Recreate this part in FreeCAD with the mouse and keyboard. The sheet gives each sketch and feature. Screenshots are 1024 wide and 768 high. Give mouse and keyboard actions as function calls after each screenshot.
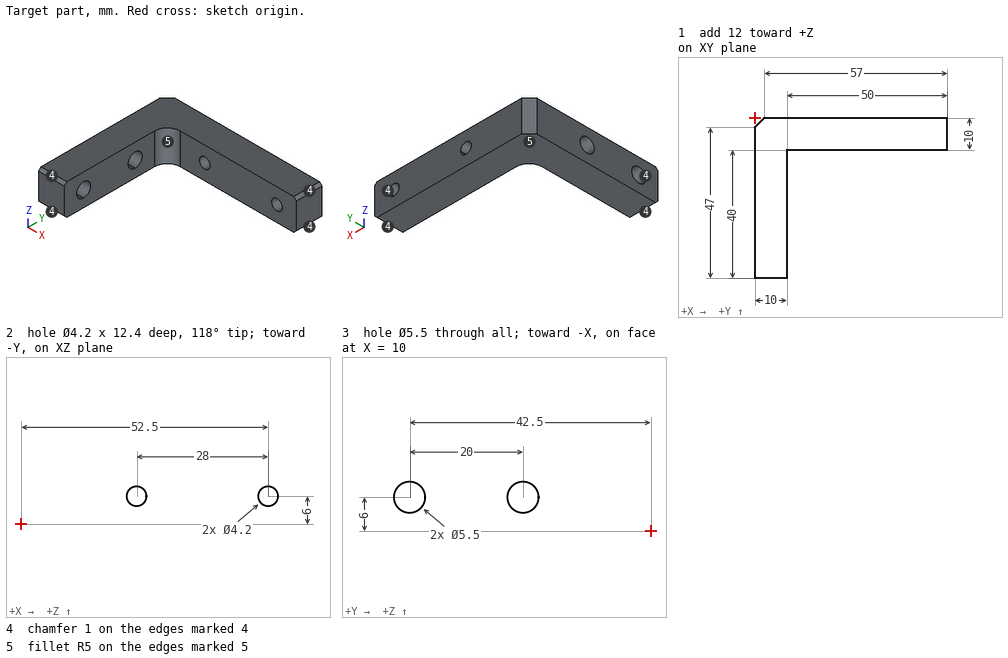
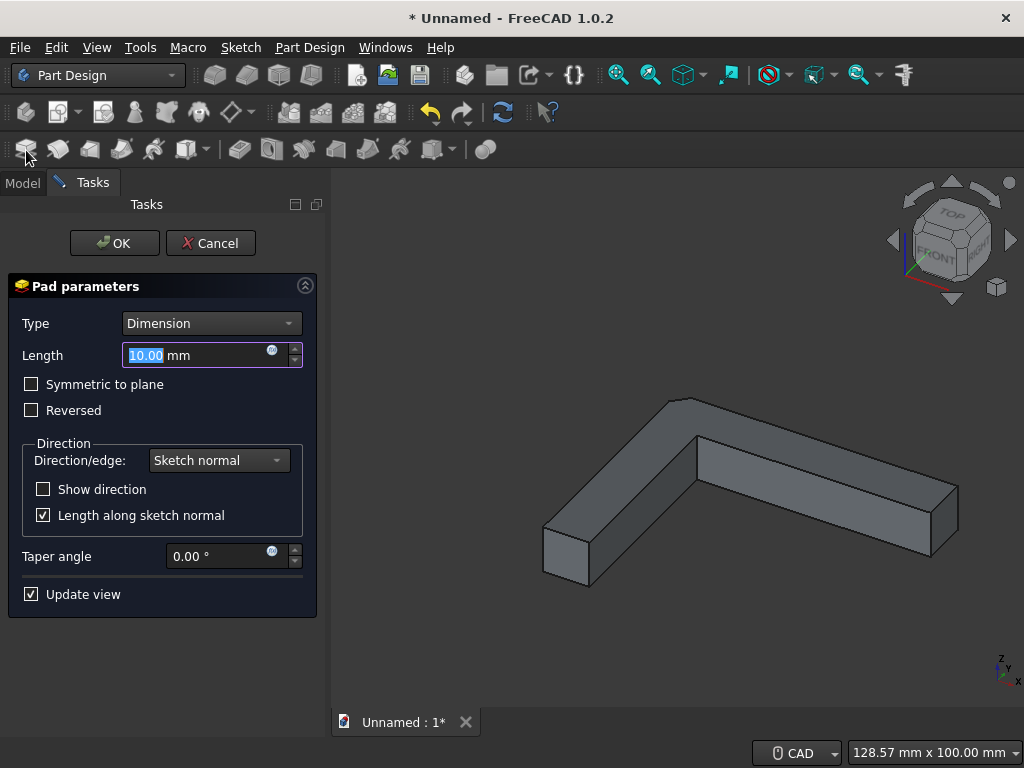
text(12)
key(Tab)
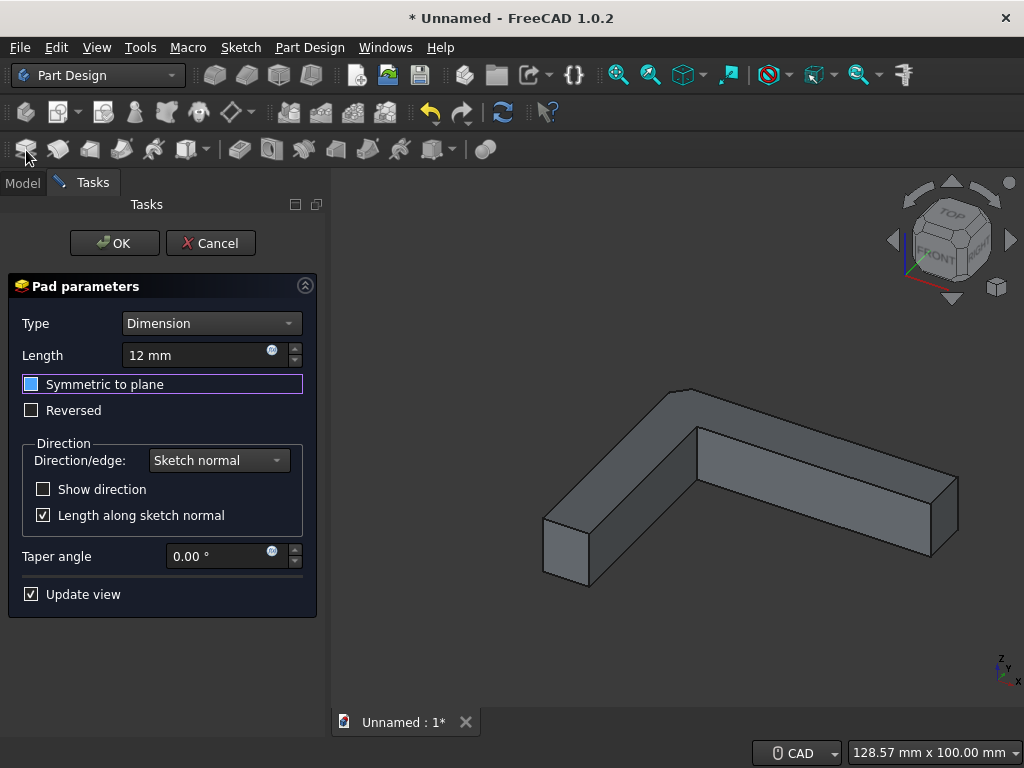
click(115, 243)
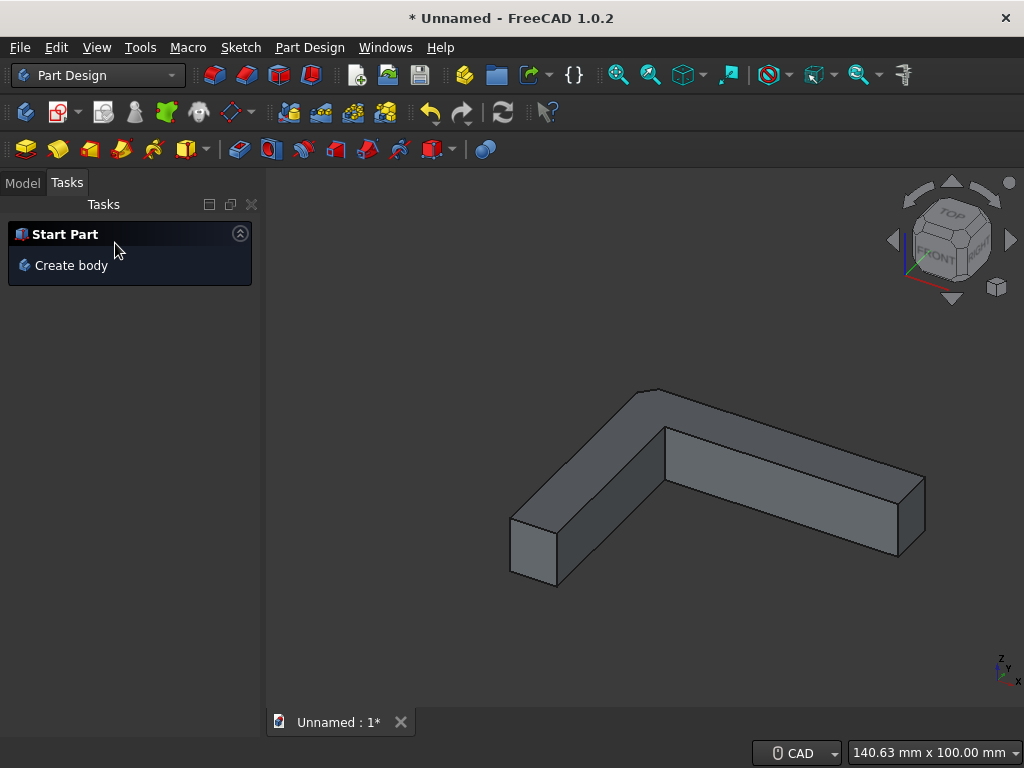
click(58, 112)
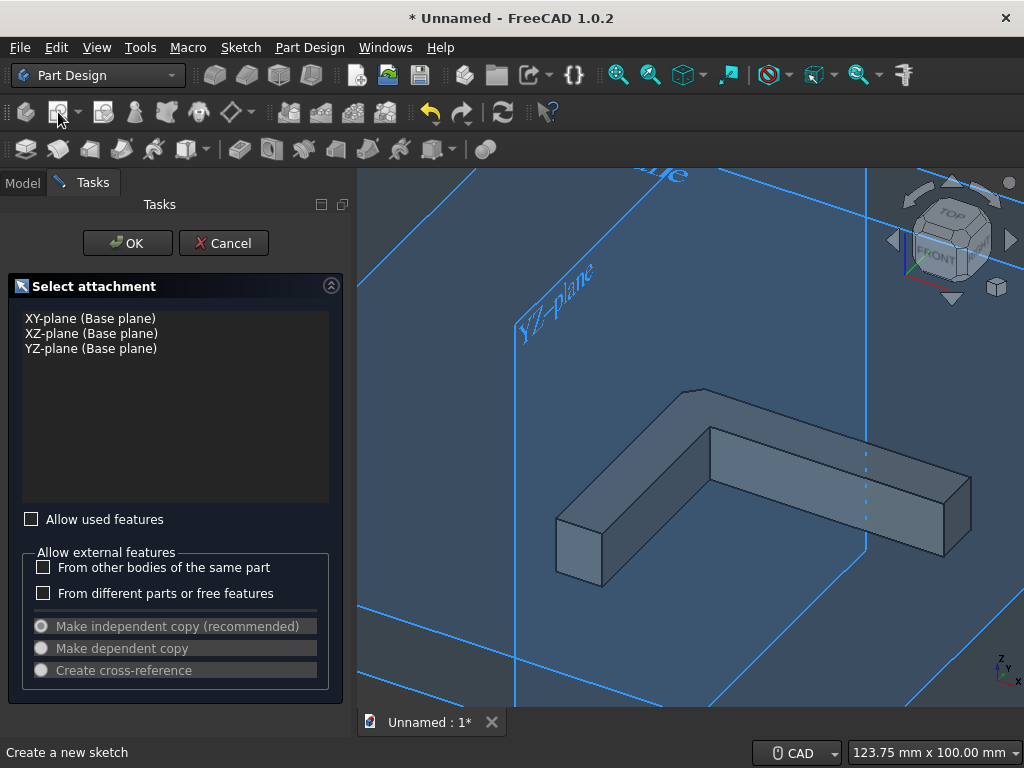
click(82, 334)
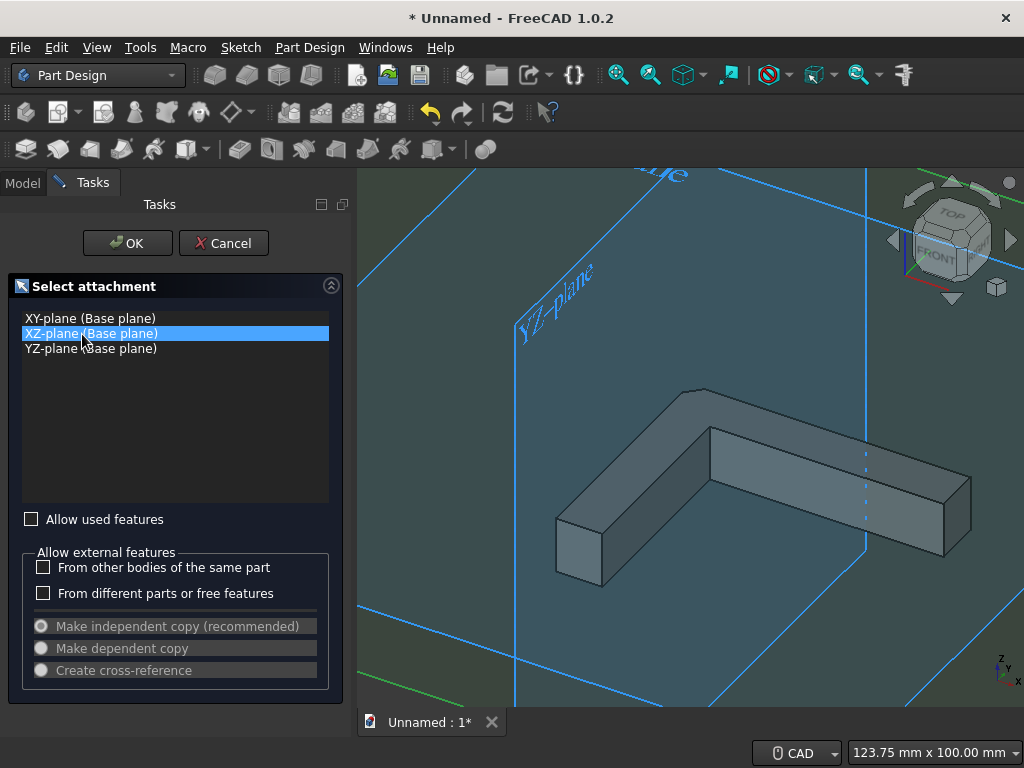
click(128, 243)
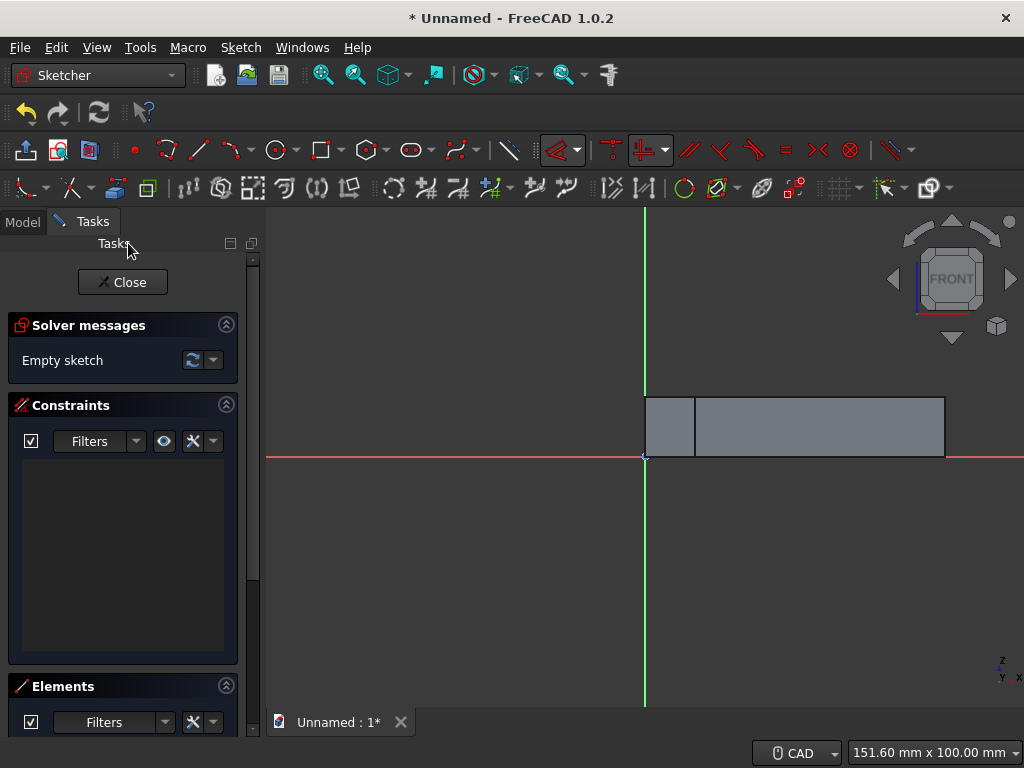
click(90, 150)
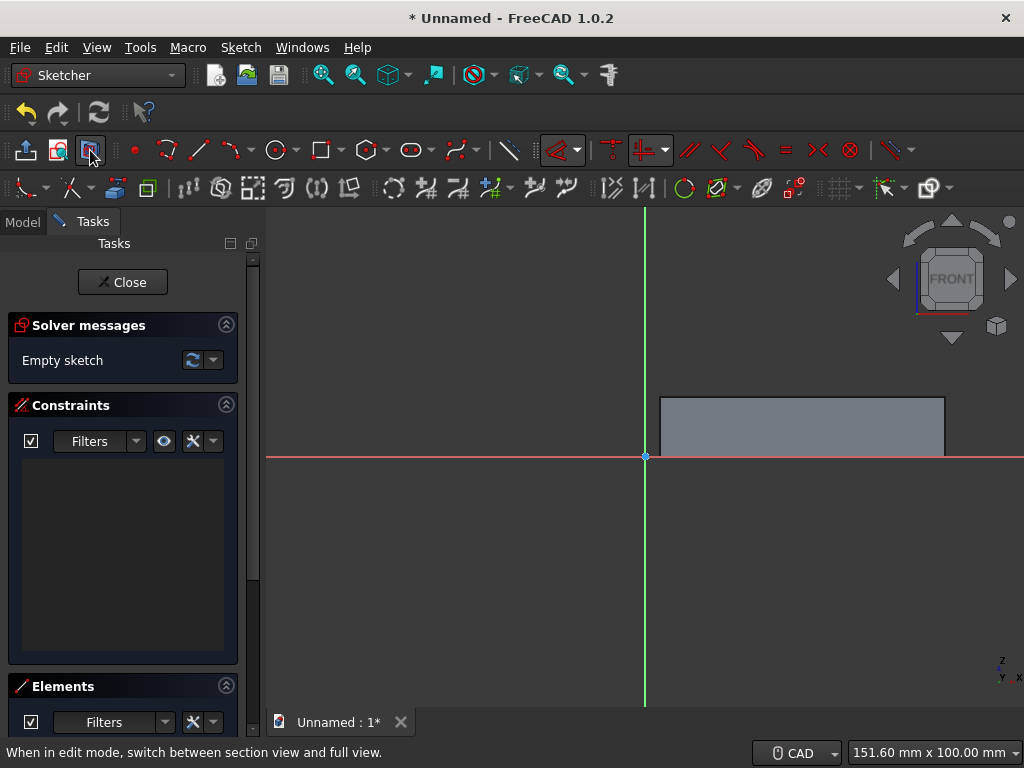
scroll(294, 548, down, 1)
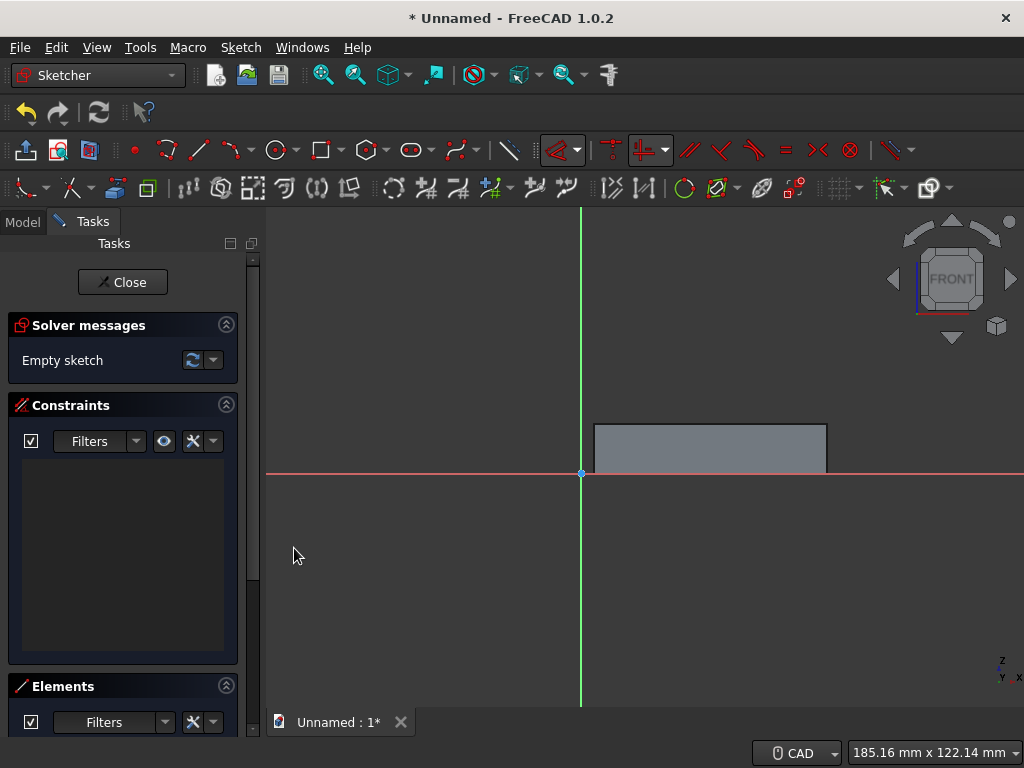
scroll(835, 457, up, 3)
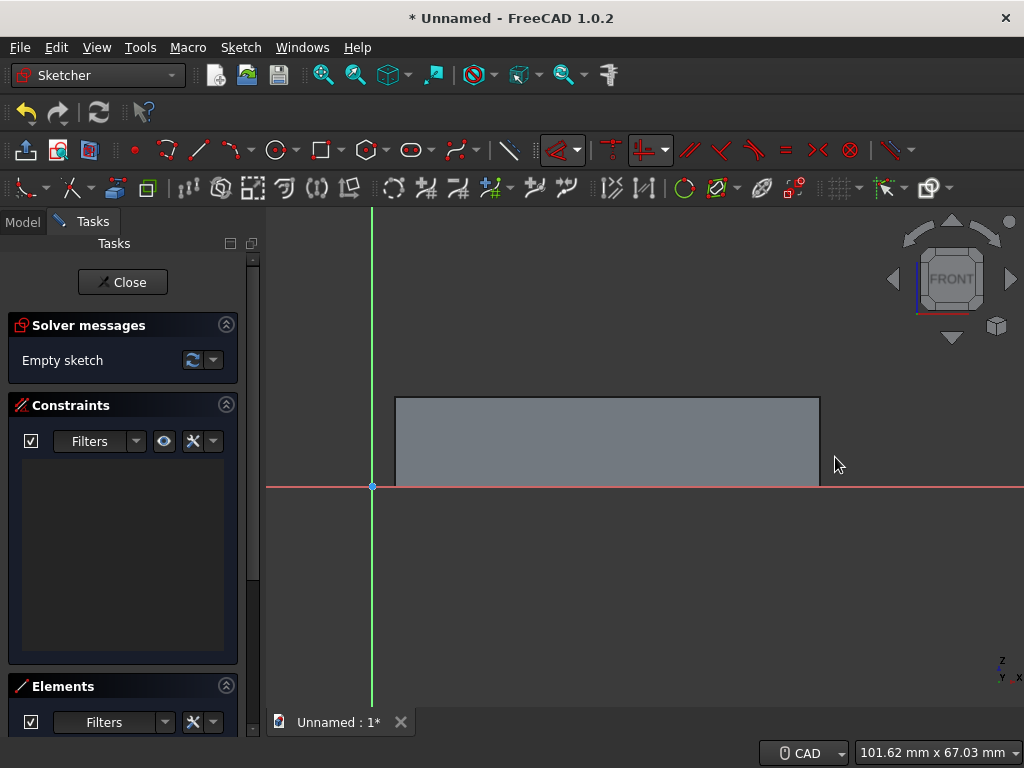
click(276, 150)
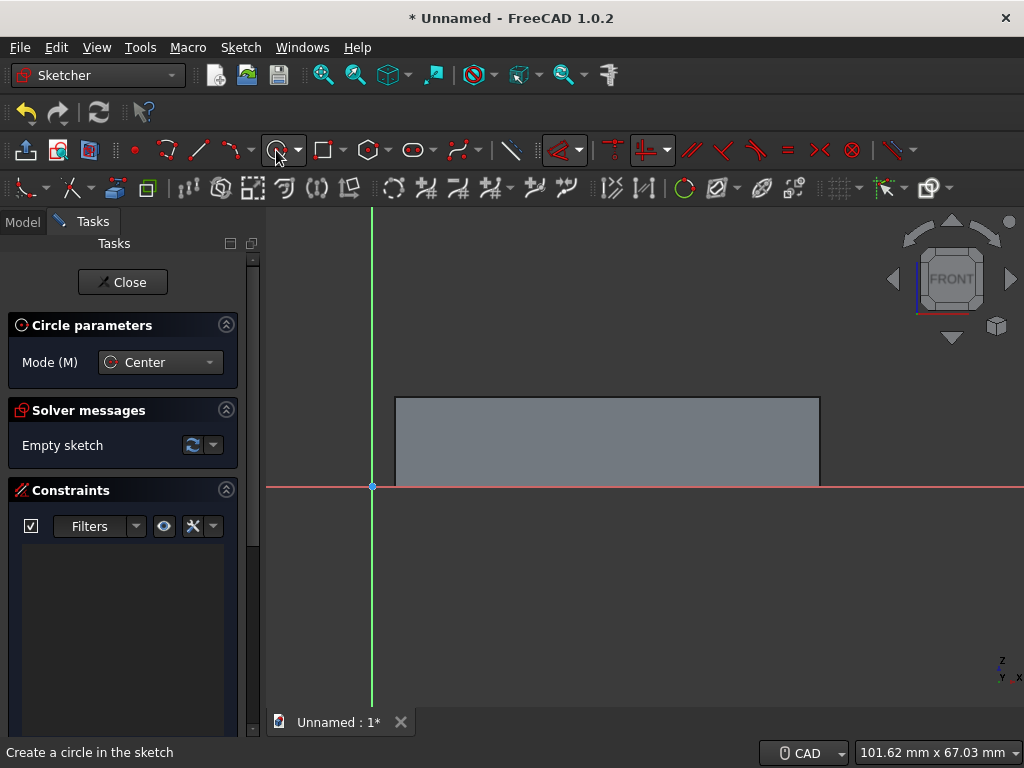
scroll(764, 442, up, 2)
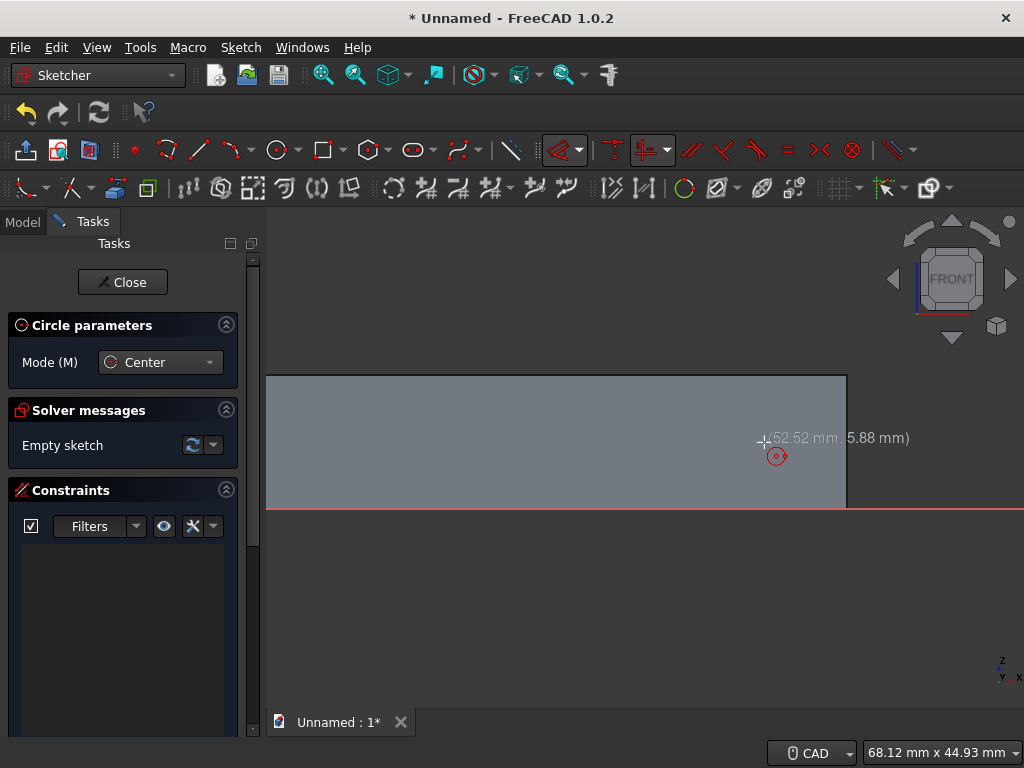
click(763, 442)
click(780, 425)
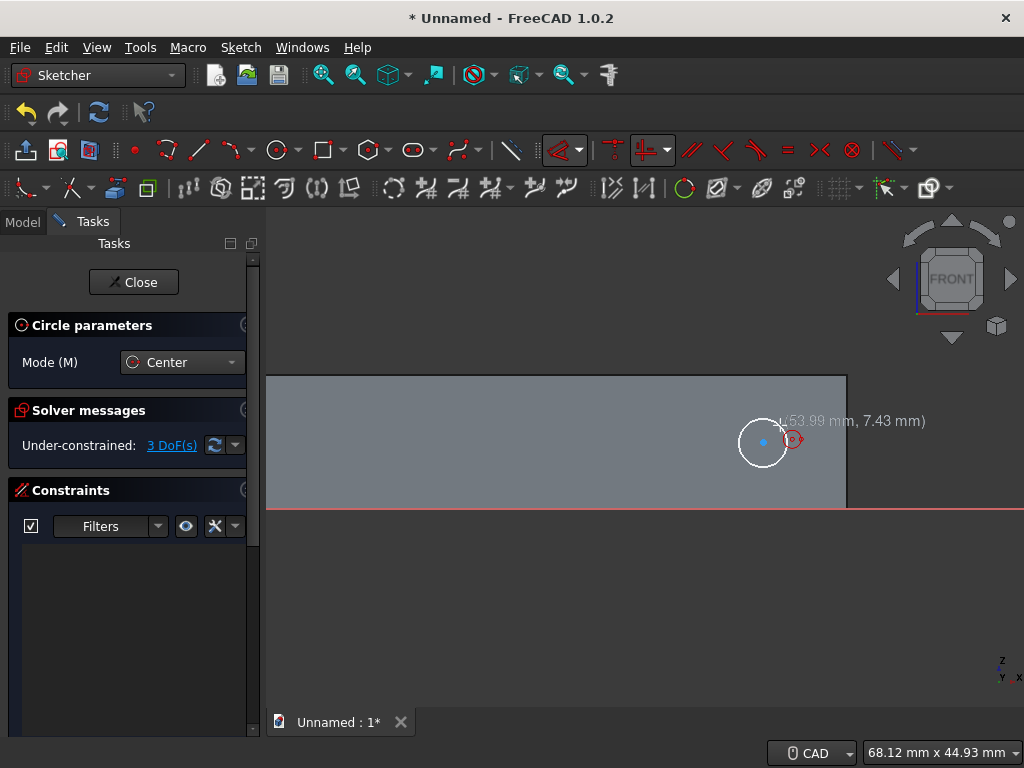
click(452, 442)
click(468, 425)
key(Escape)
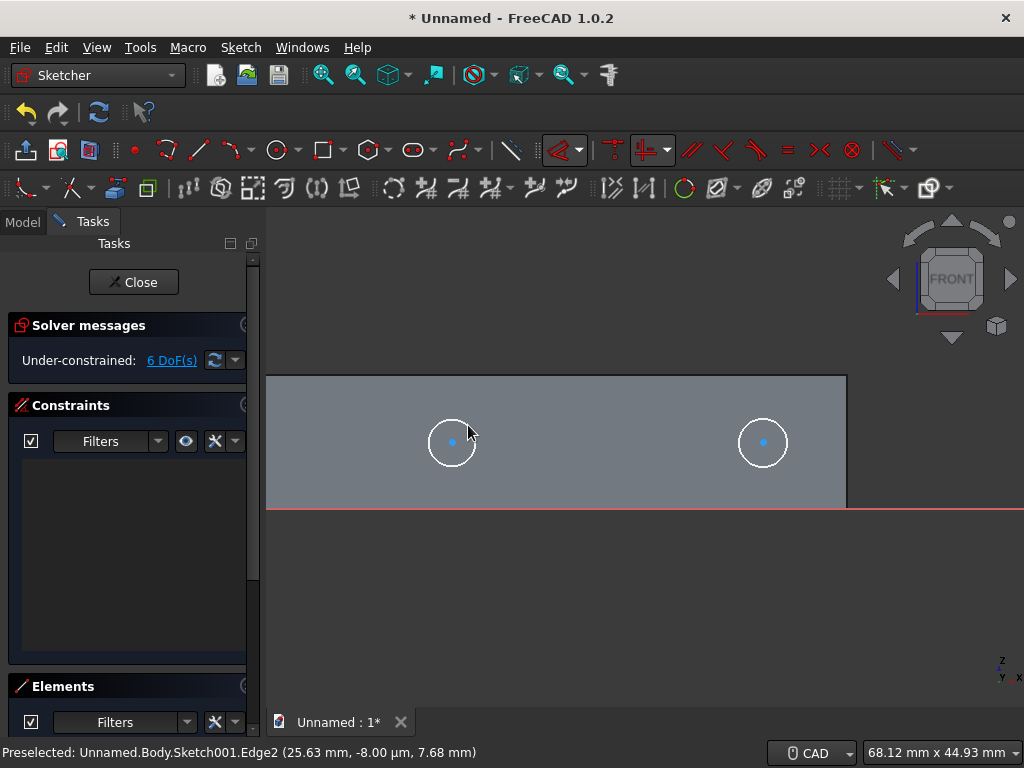
click(780, 426)